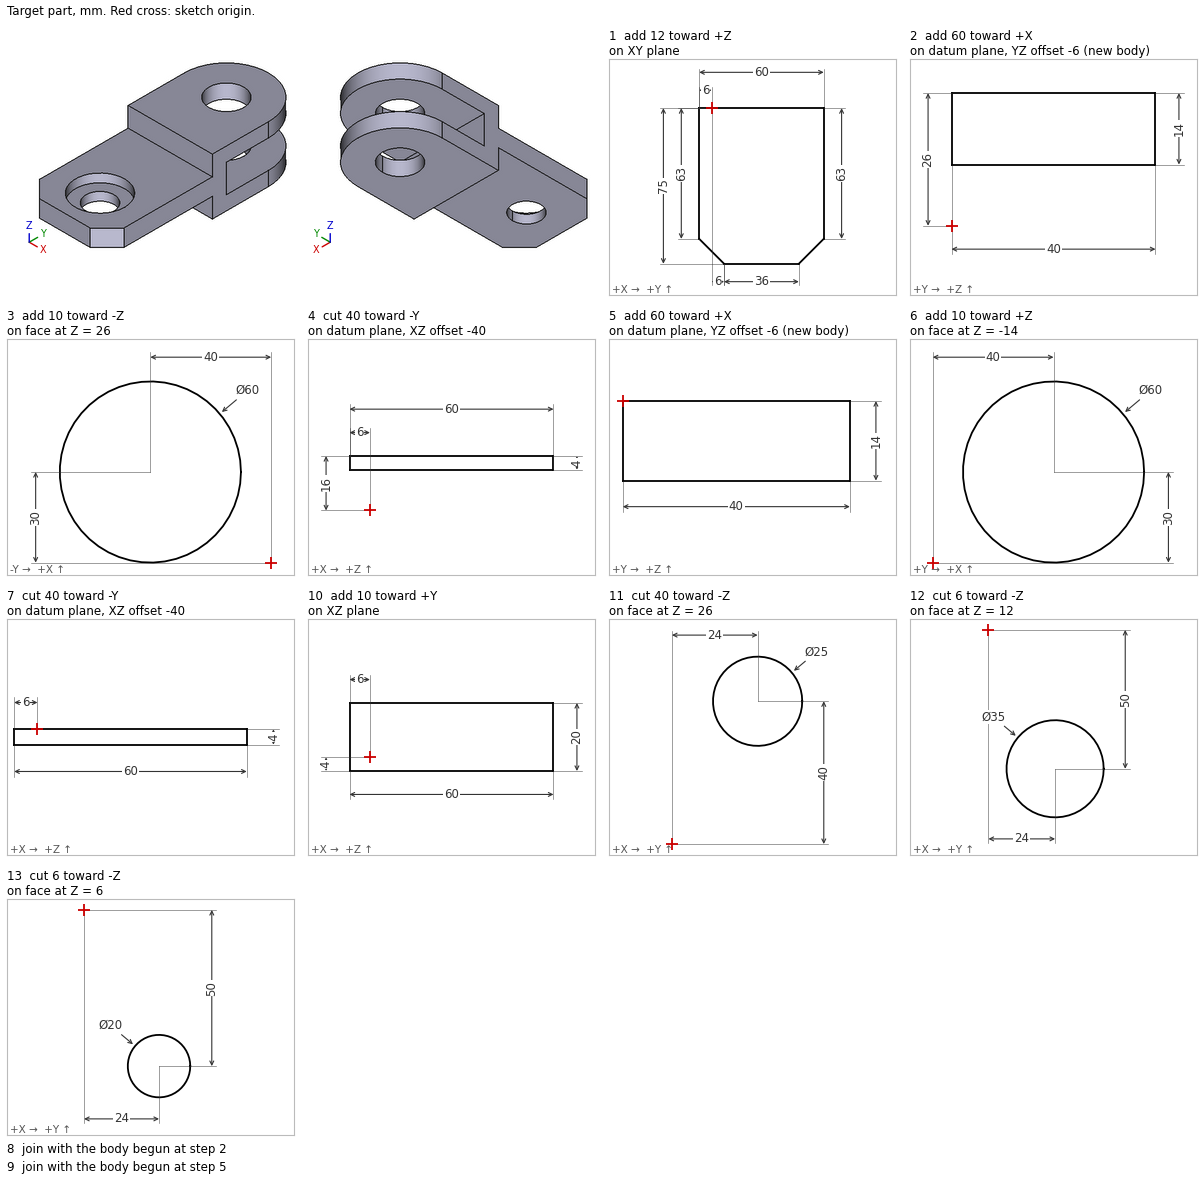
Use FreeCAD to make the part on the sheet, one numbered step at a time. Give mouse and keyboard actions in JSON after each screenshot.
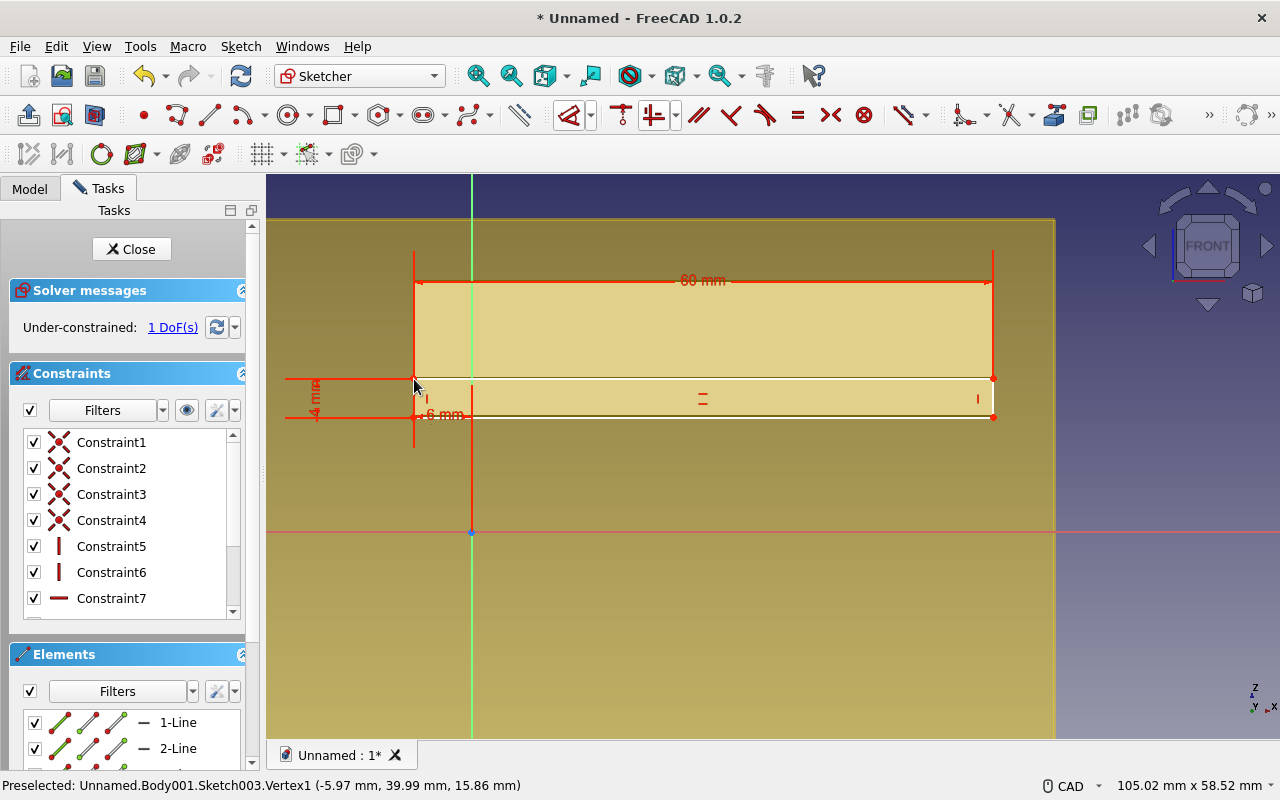
{"action": "left_click", "coordinate": [414, 379]}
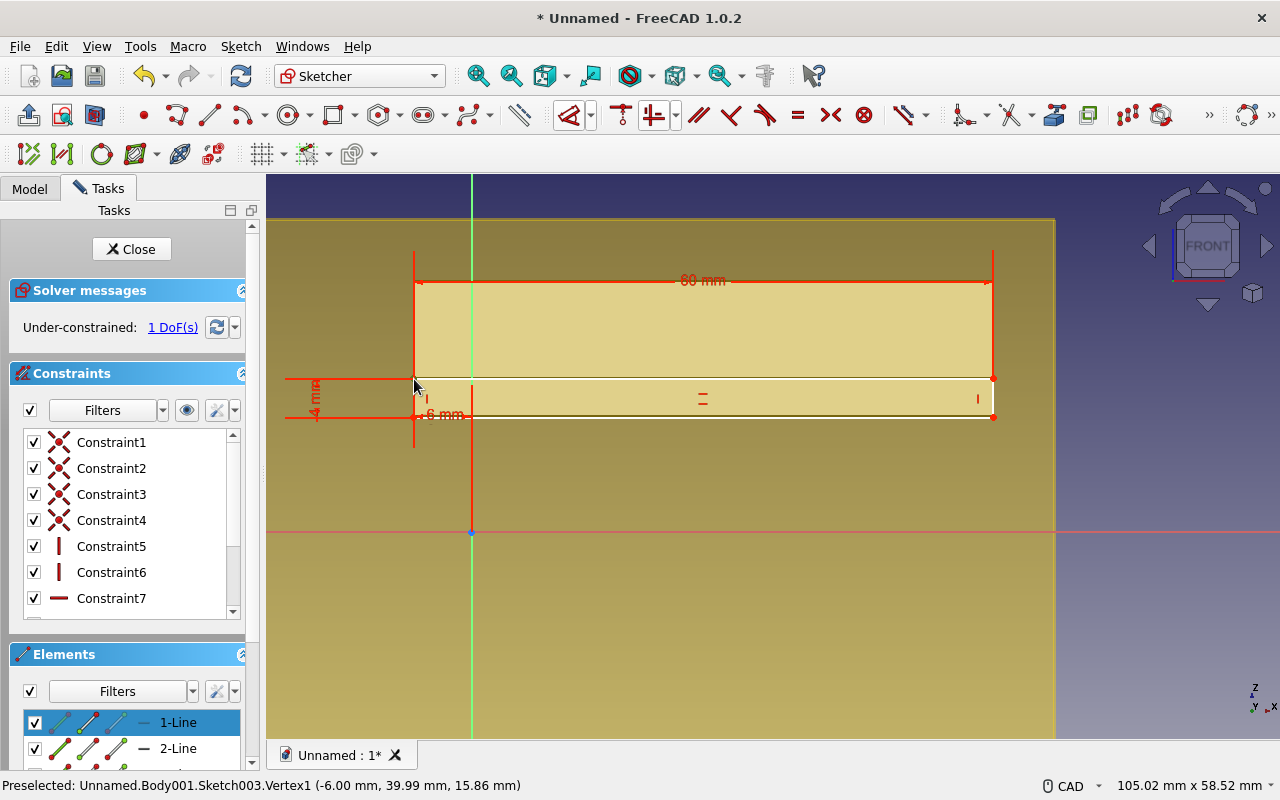
{"action": "left_click", "coordinate": [590, 116]}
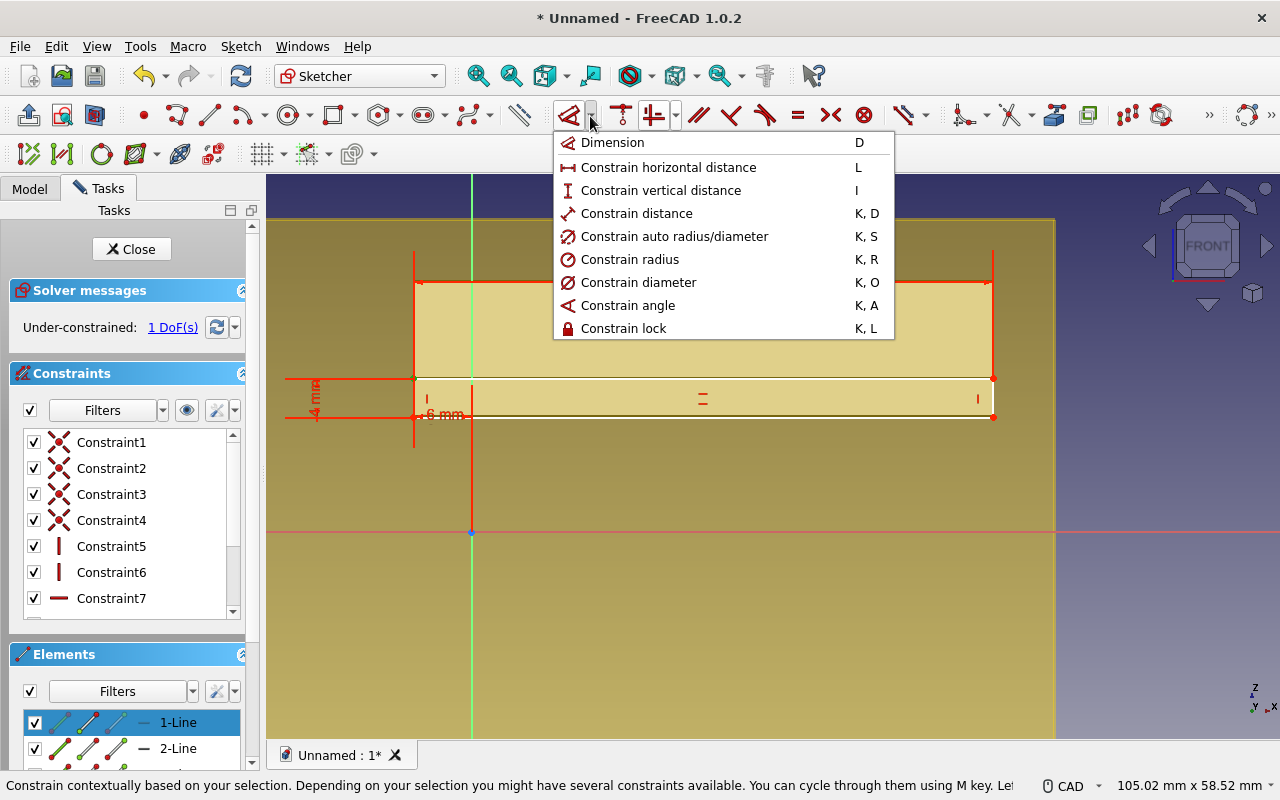
{"action": "left_click", "coordinate": [724, 190]}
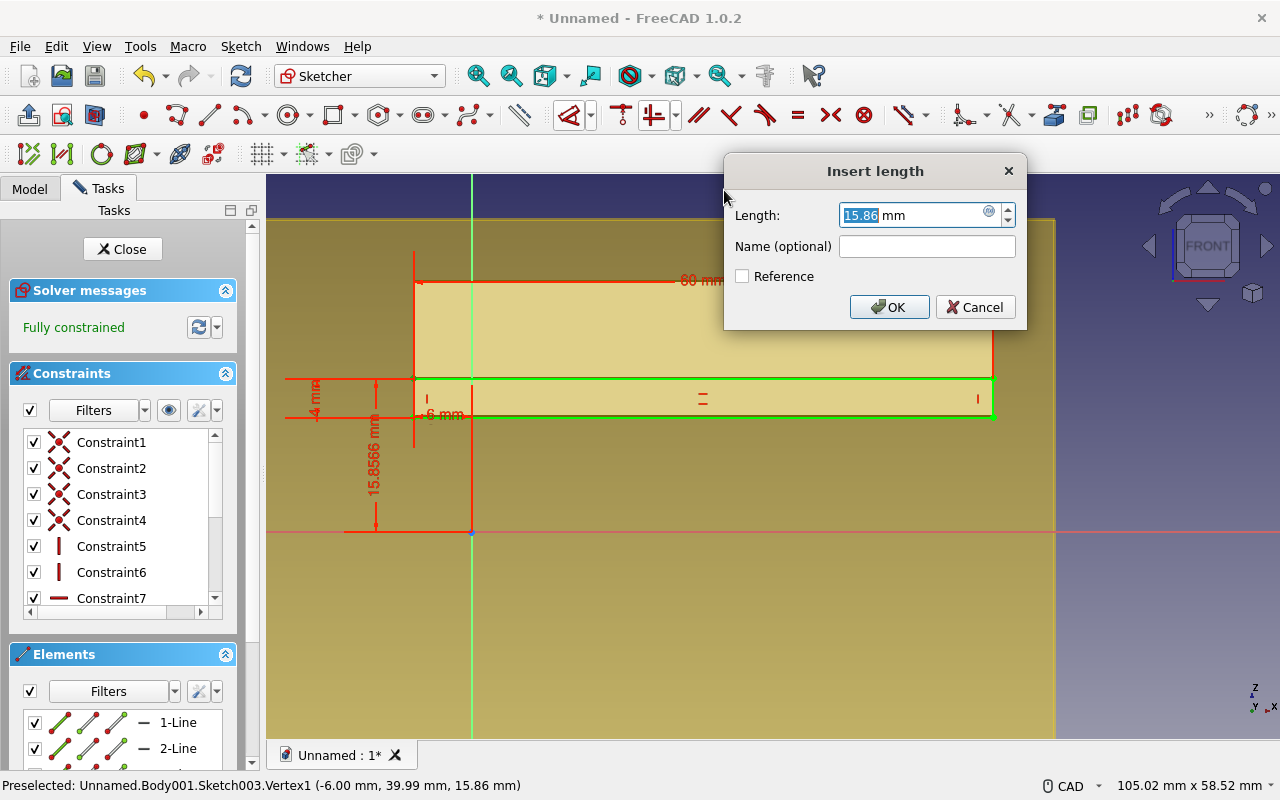
{"action": "type", "text": "16"}
{"action": "key", "text": "Return"}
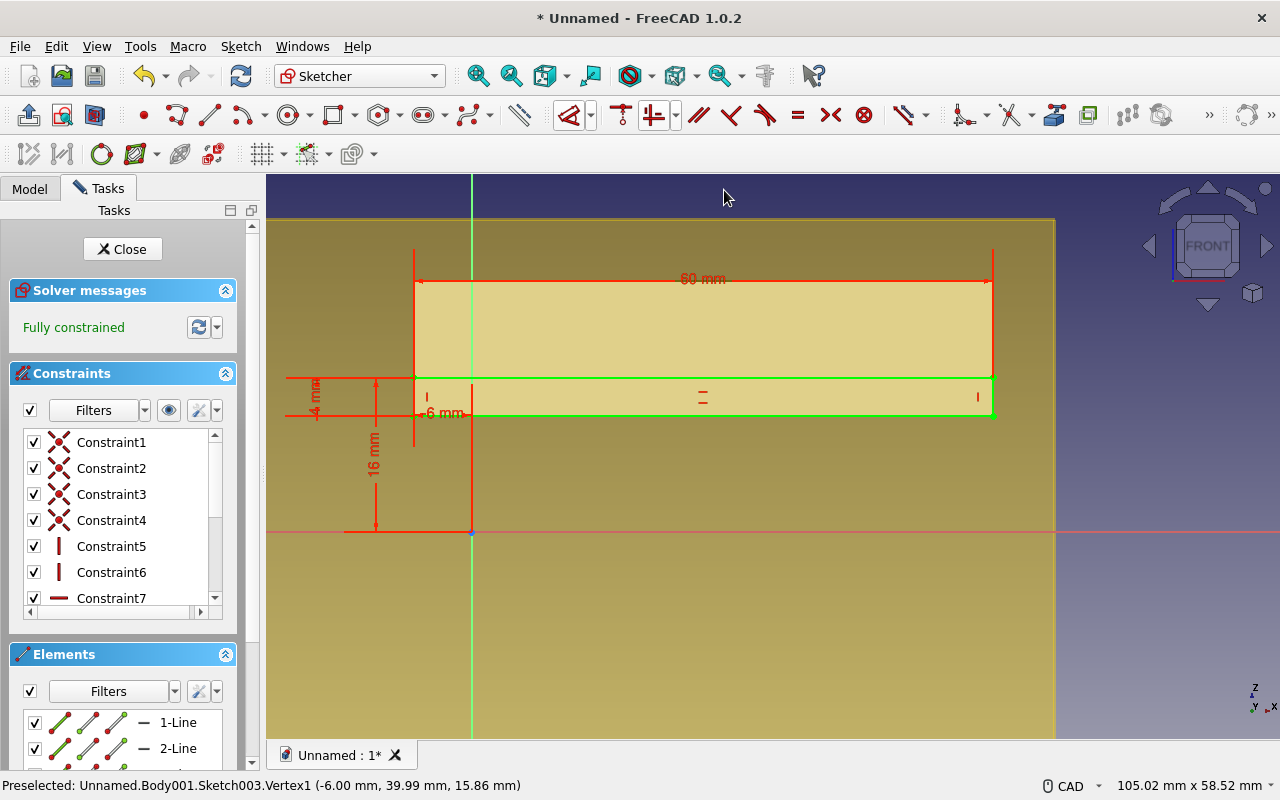
{"action": "left_click", "coordinate": [123, 249]}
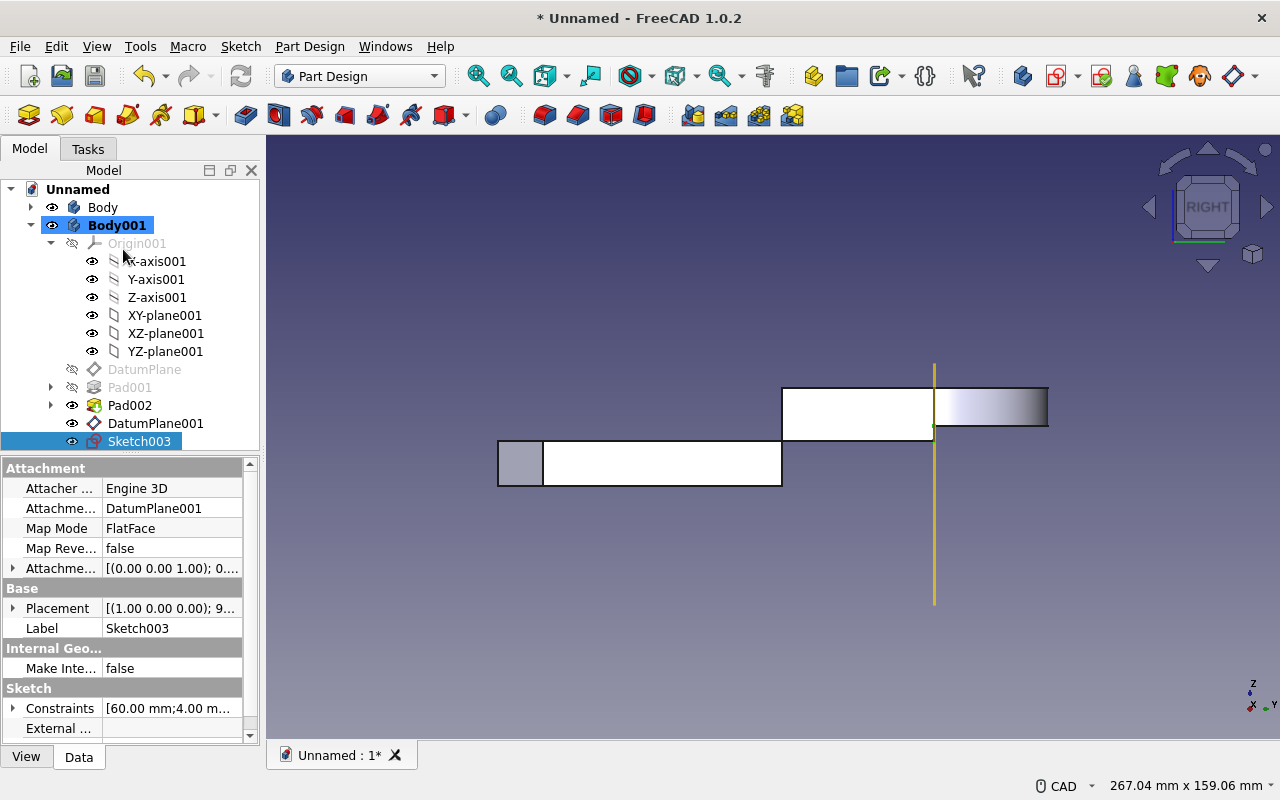
{"action": "left_click", "coordinate": [246, 116]}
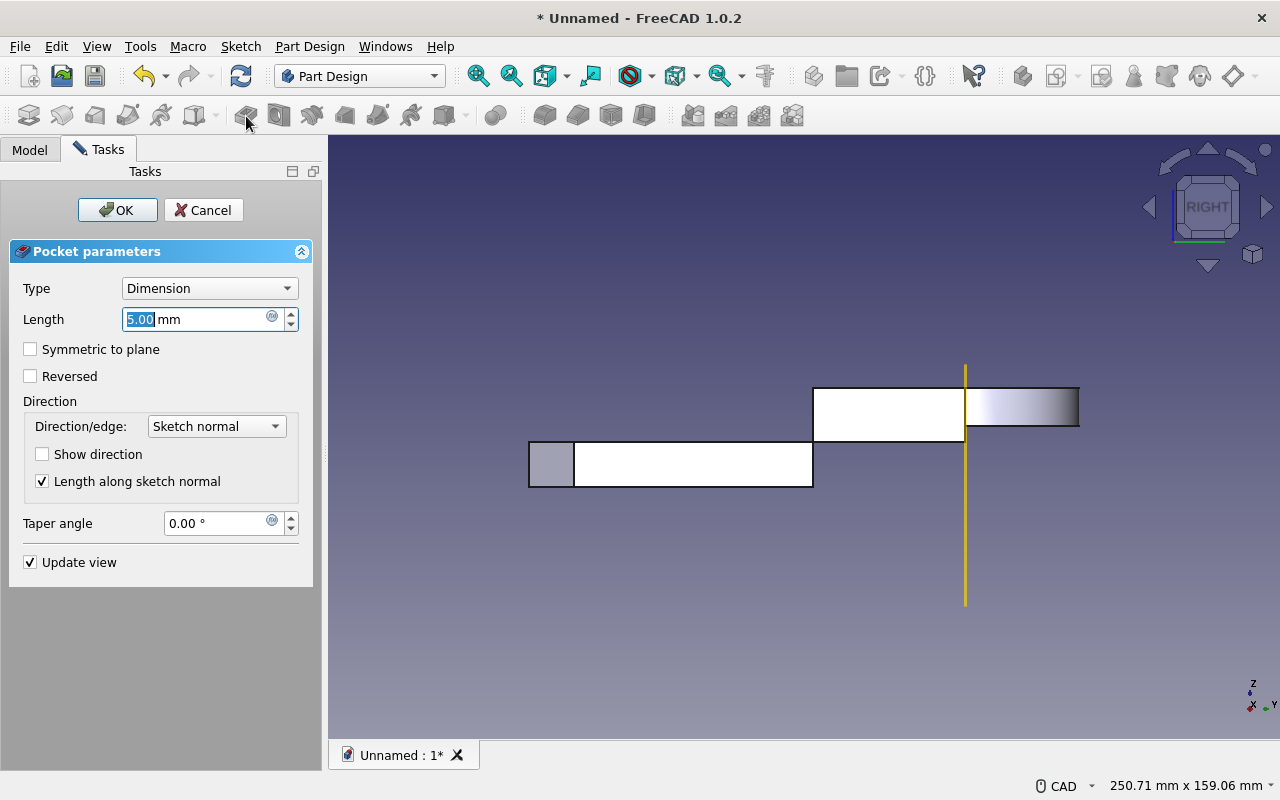
{"action": "type", "text": "40"}
{"action": "key", "text": "Tab"}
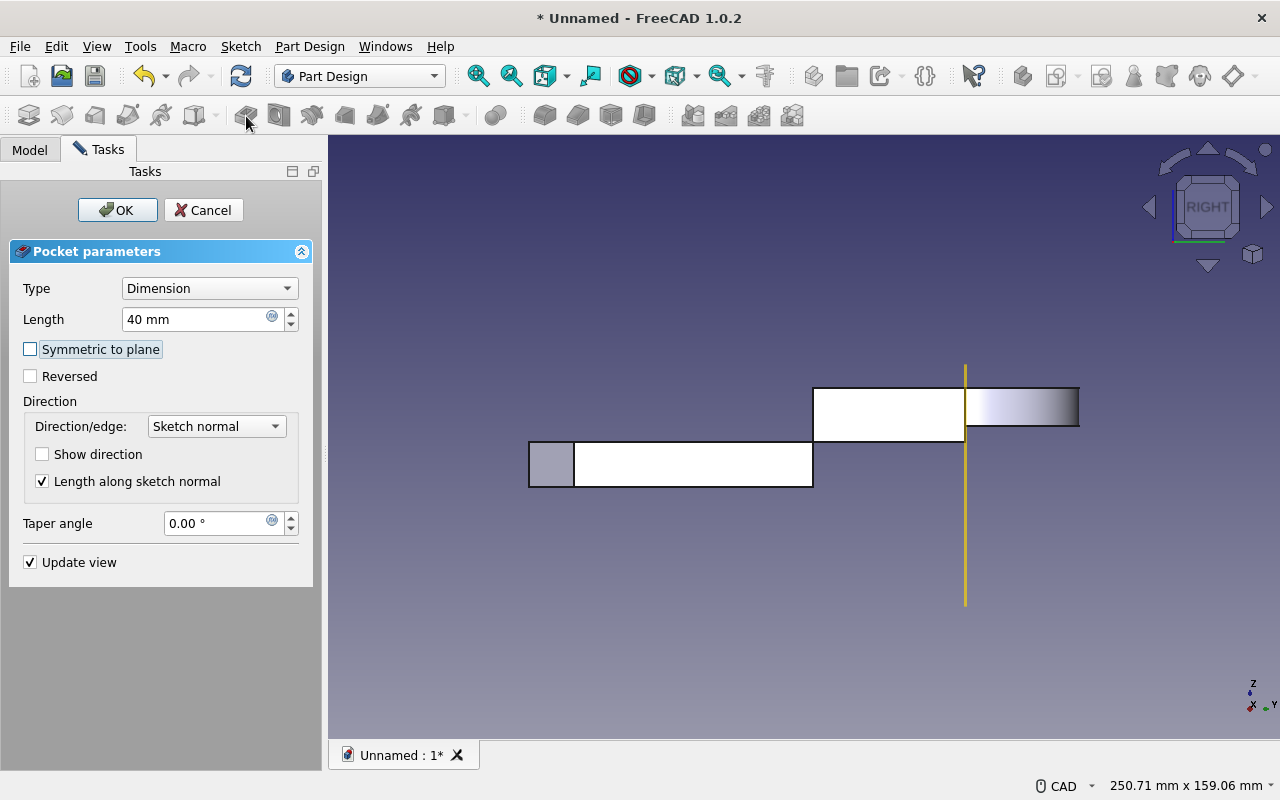
{"action": "left_click", "coordinate": [31, 376]}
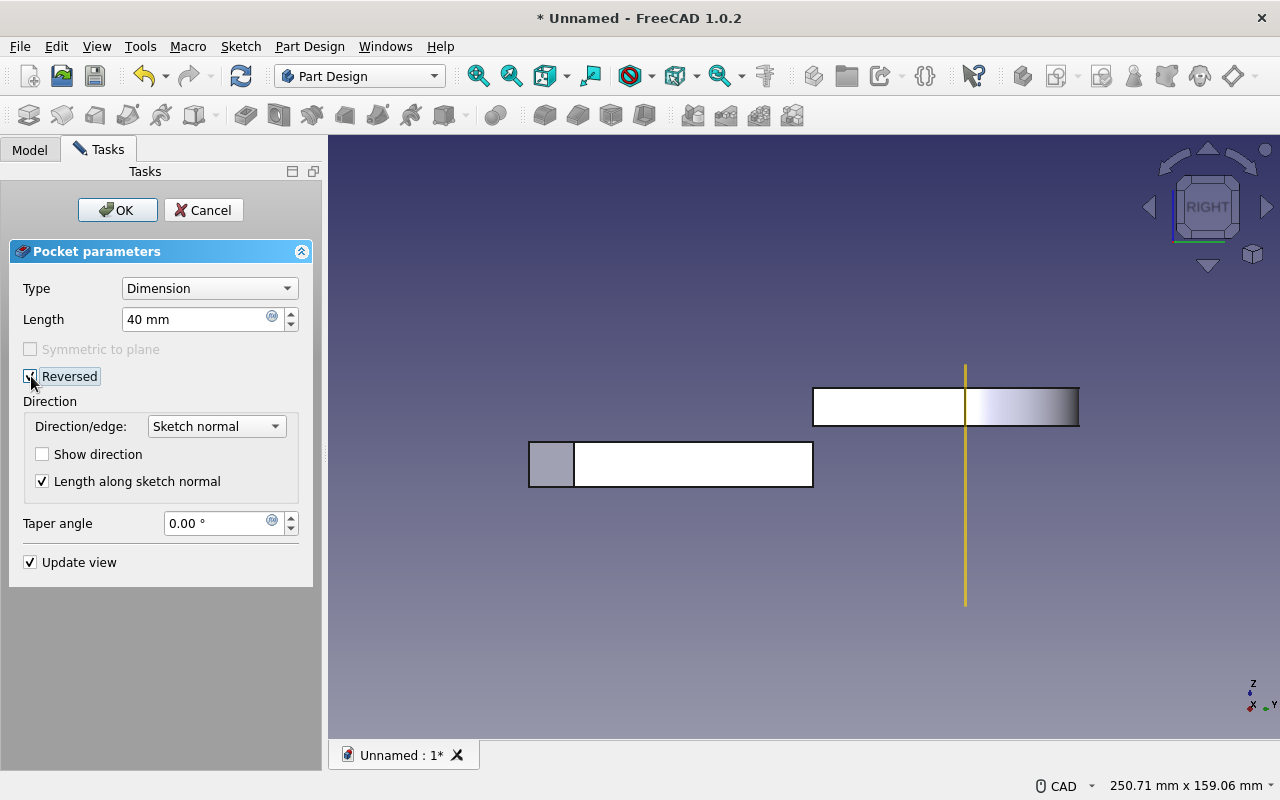
{"action": "left_click", "coordinate": [118, 210]}